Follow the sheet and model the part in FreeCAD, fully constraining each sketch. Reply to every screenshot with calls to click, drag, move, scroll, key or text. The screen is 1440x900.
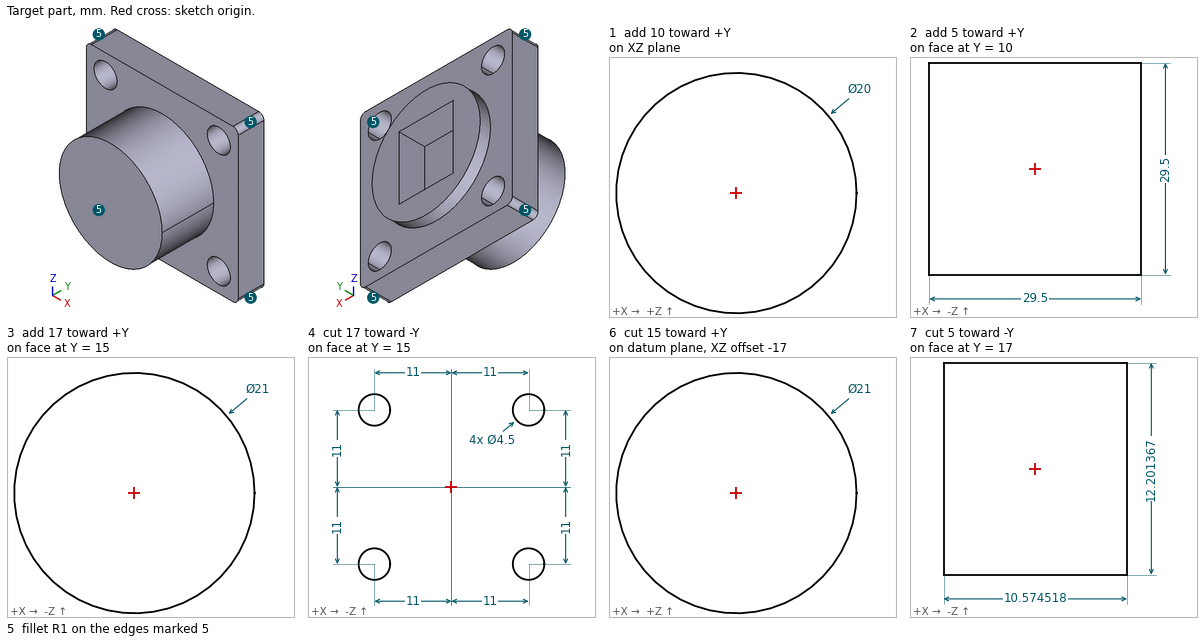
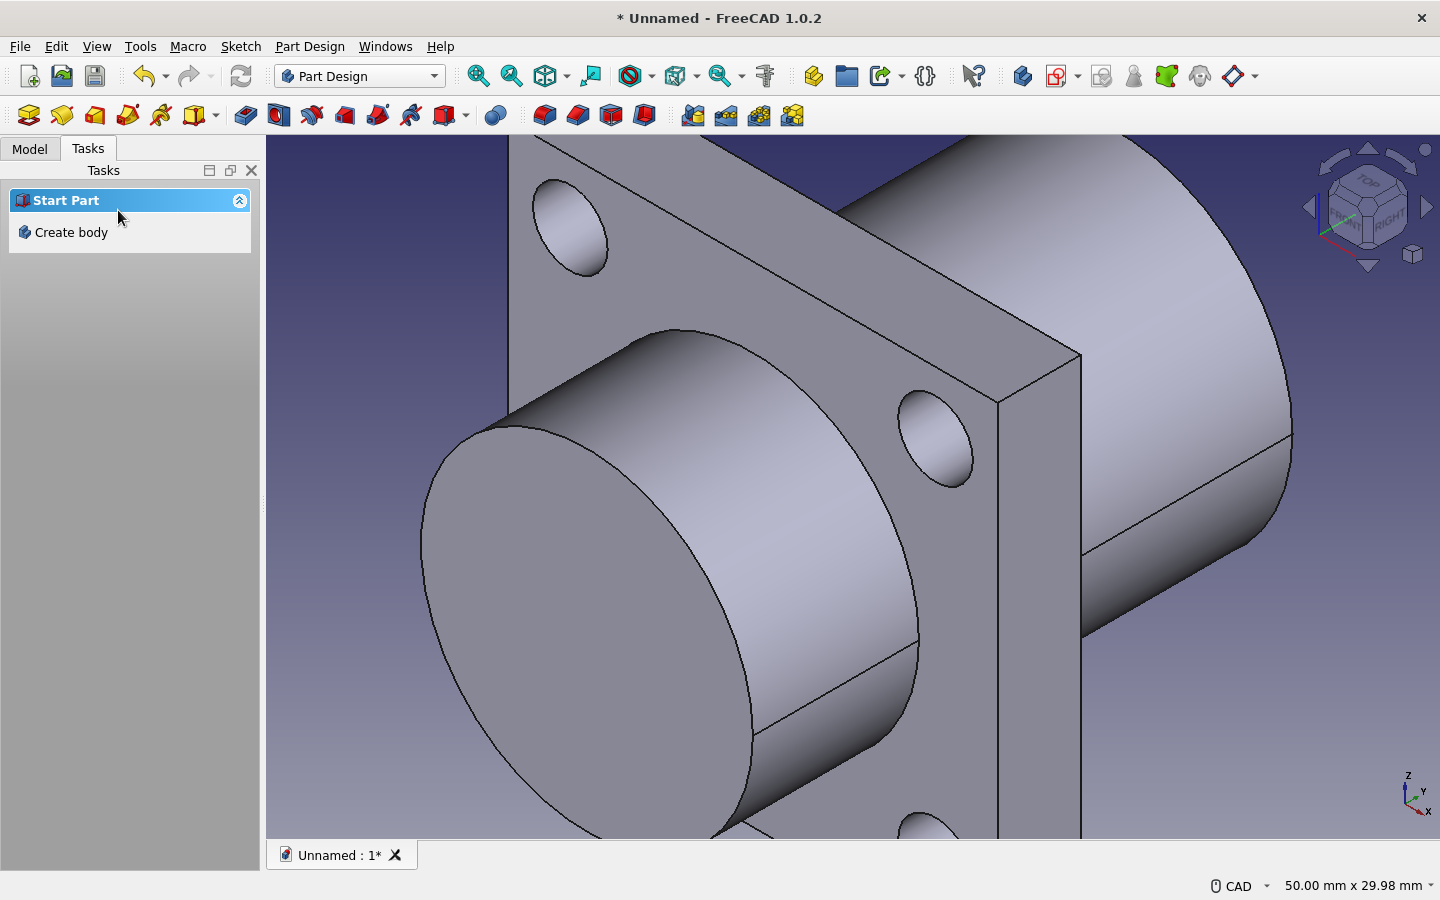
key(v)
key(f)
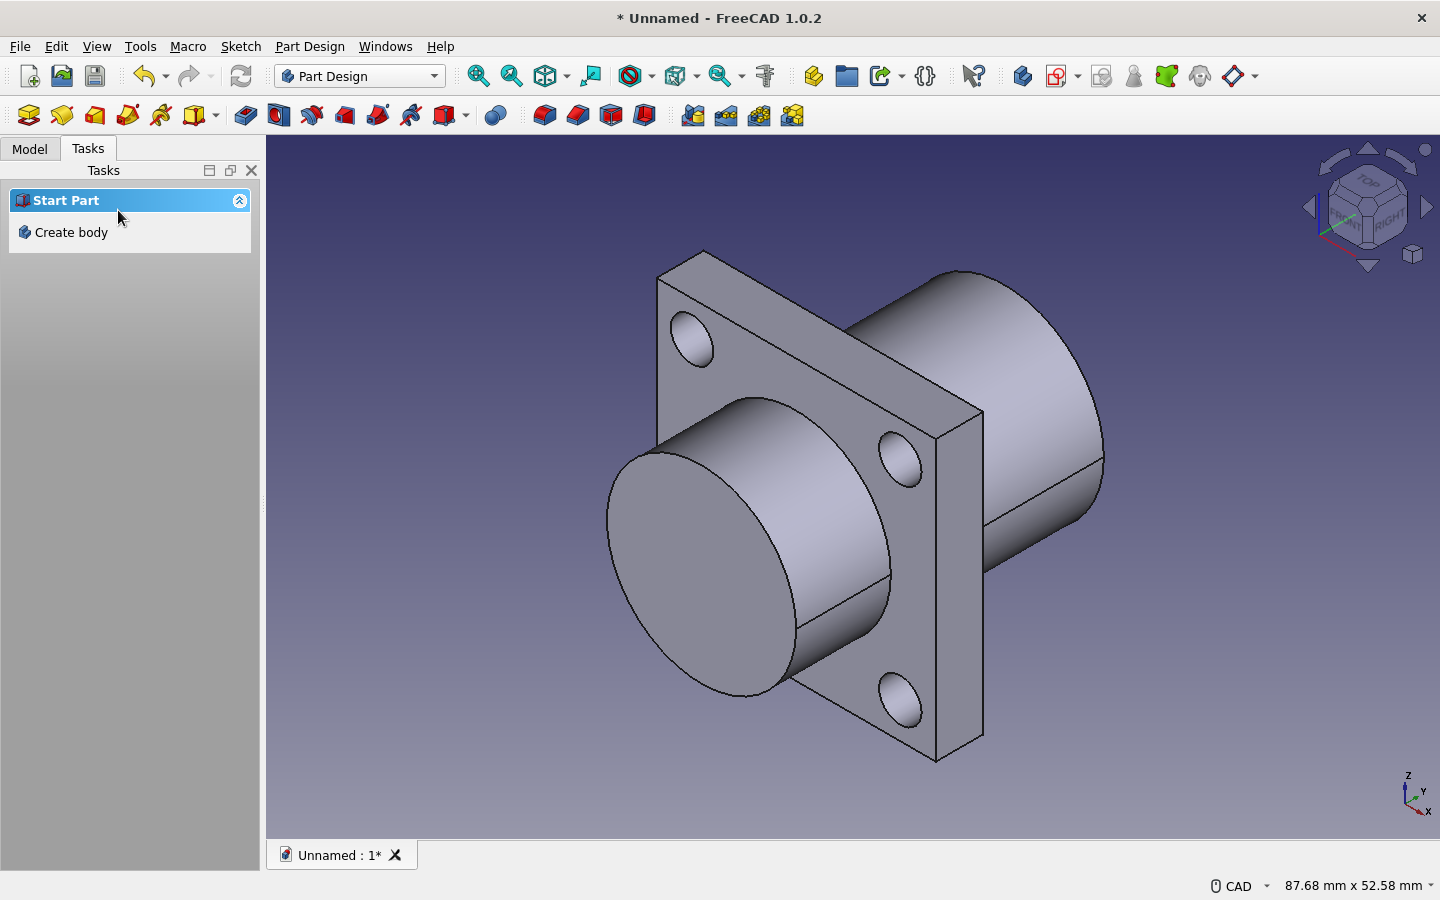
click(960, 425)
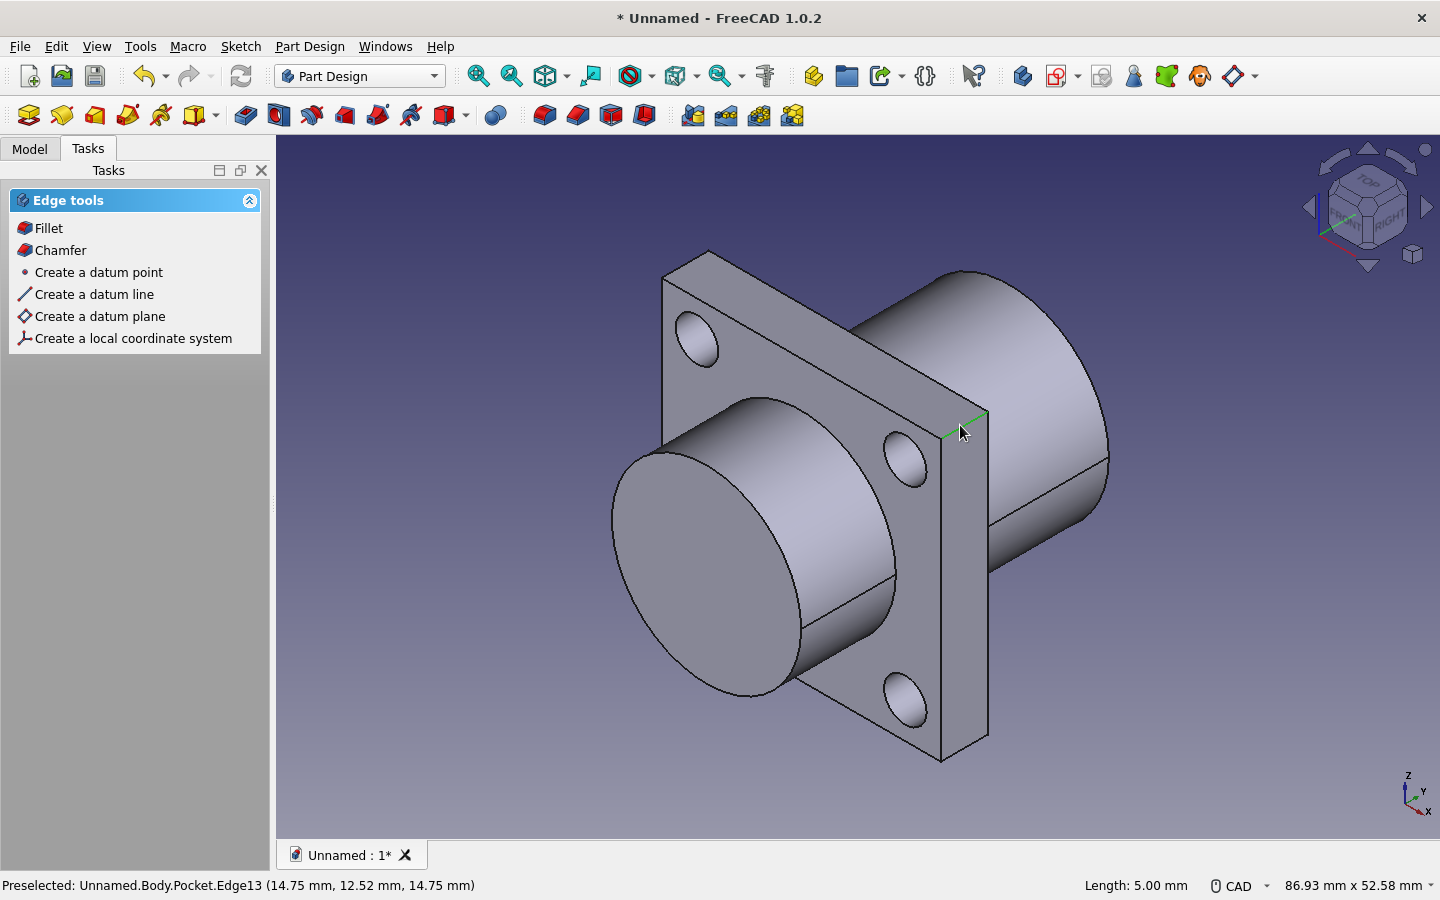
key(2)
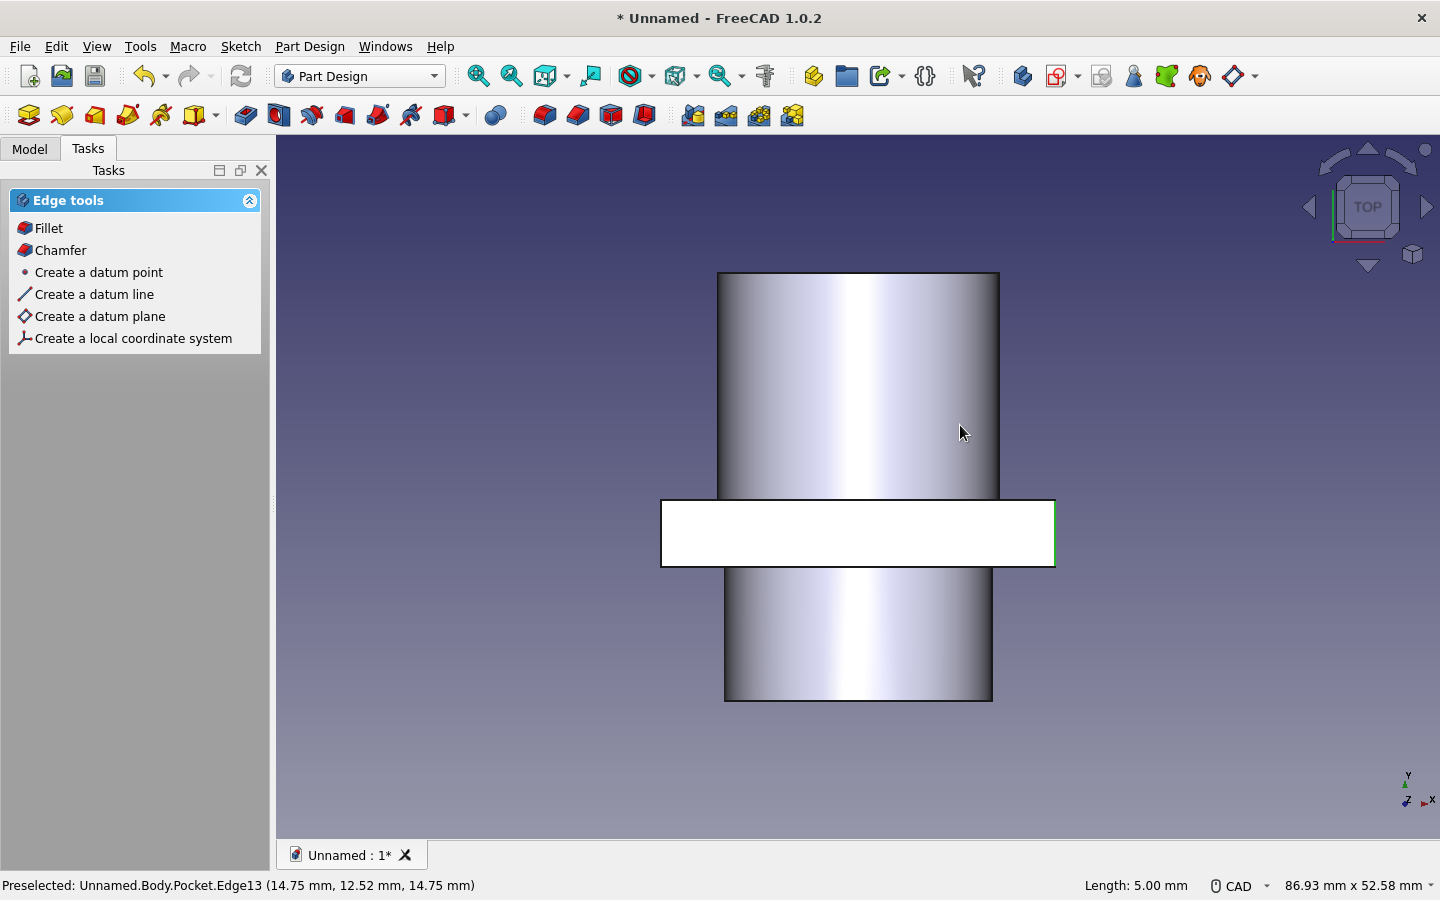
click(661, 533, ctrl)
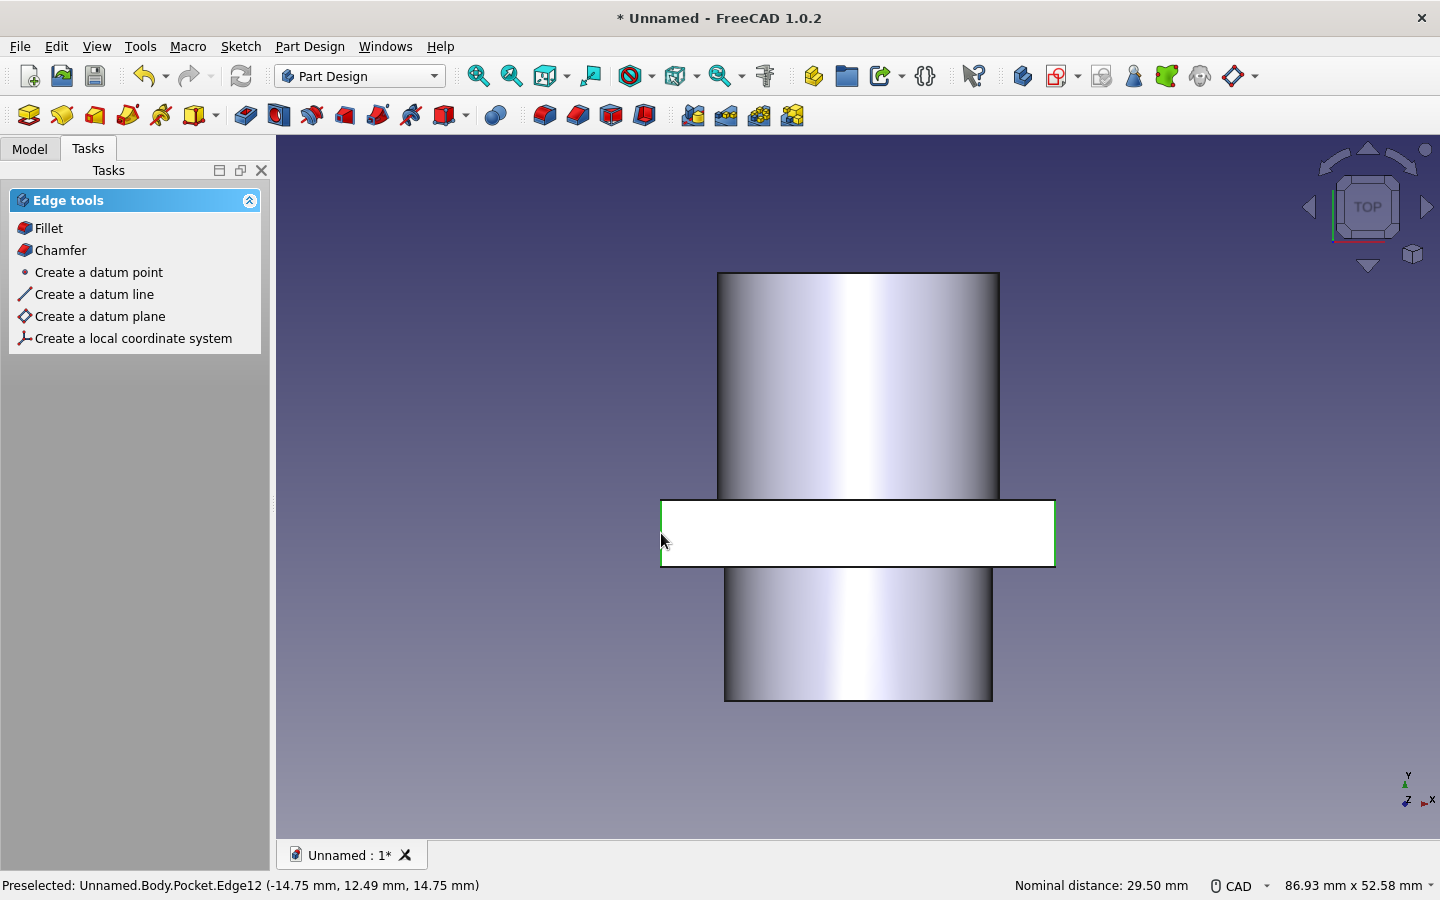
key(1)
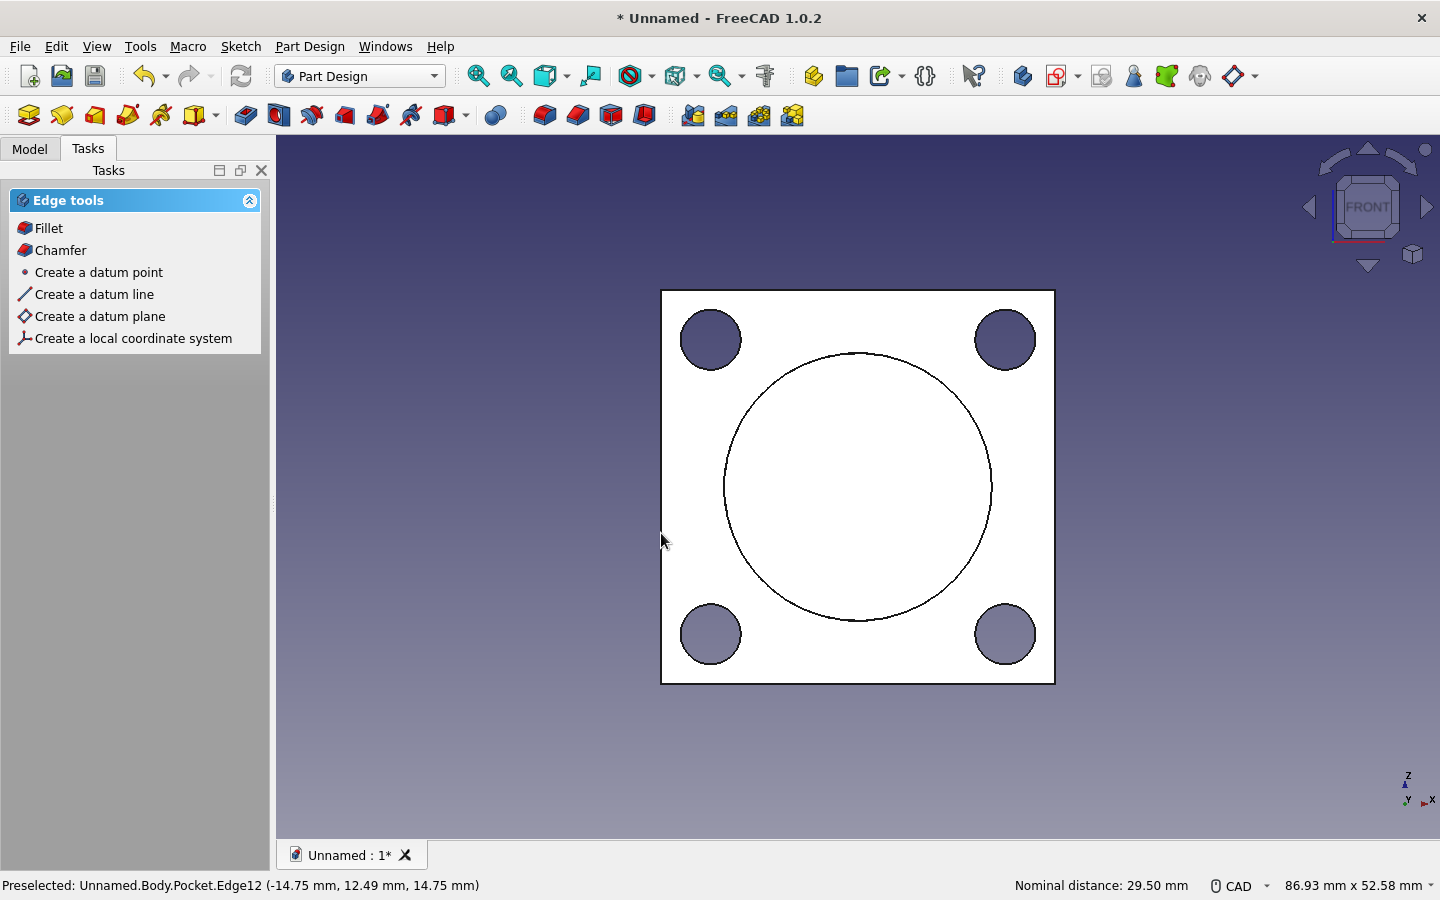
key(3)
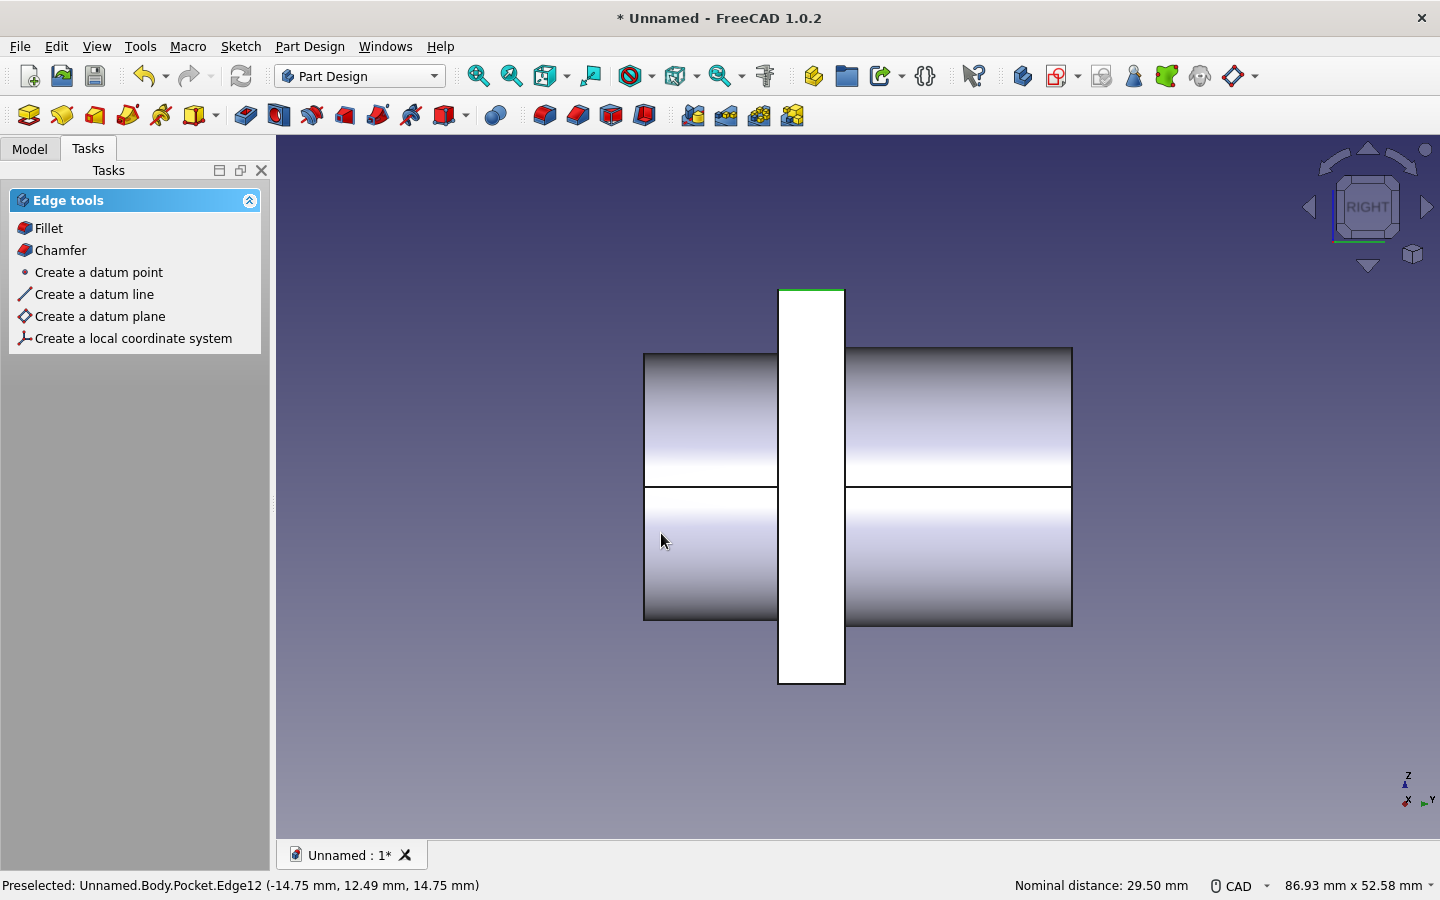
click(811, 683, ctrl)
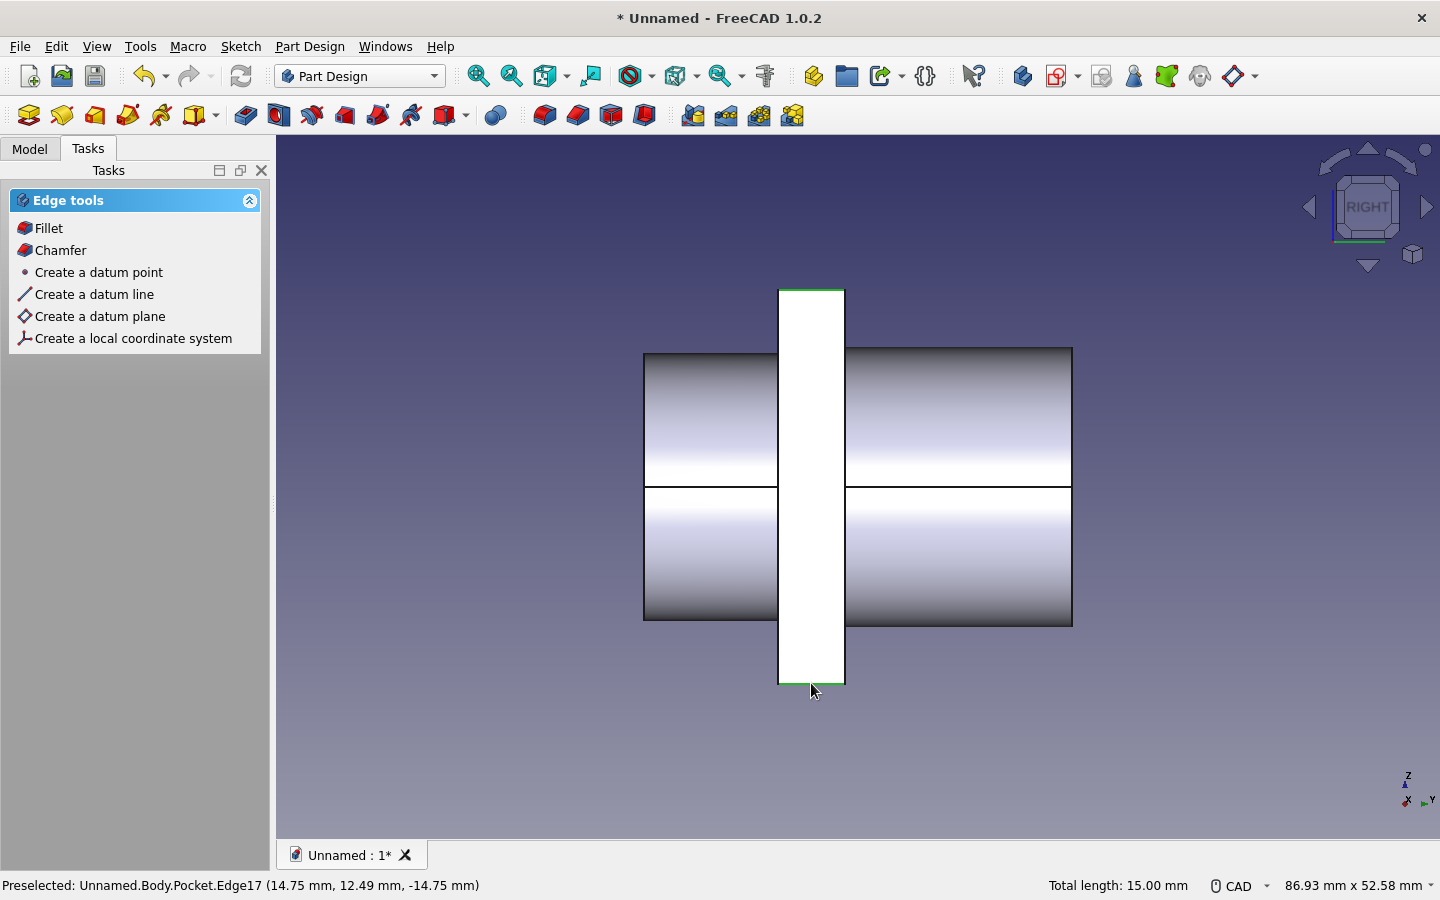
key(5)